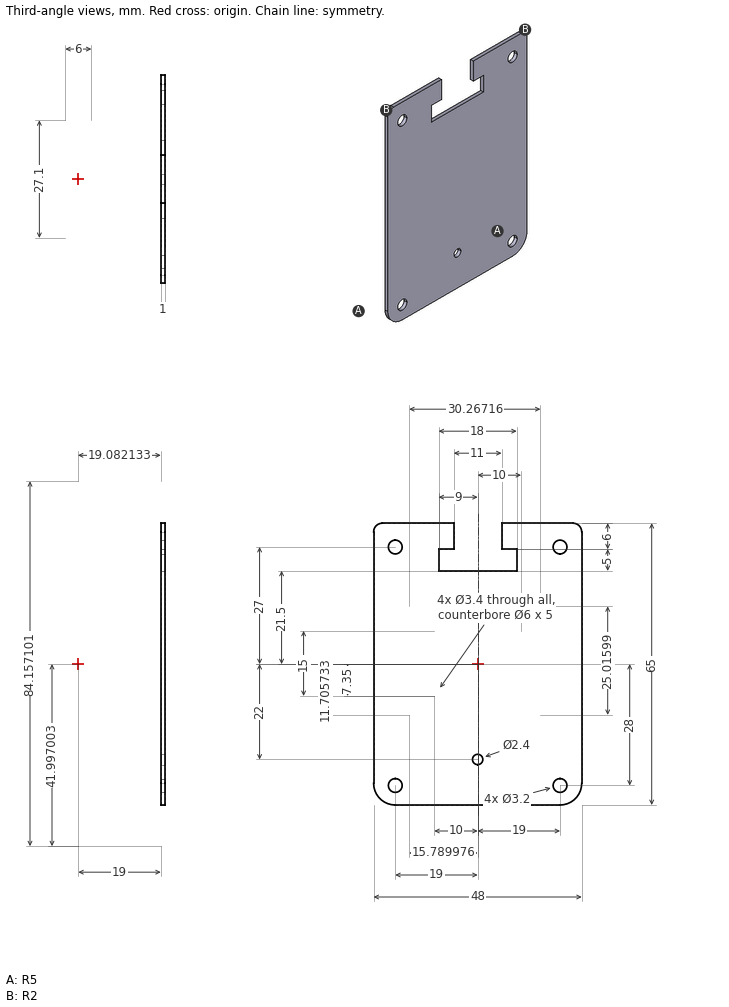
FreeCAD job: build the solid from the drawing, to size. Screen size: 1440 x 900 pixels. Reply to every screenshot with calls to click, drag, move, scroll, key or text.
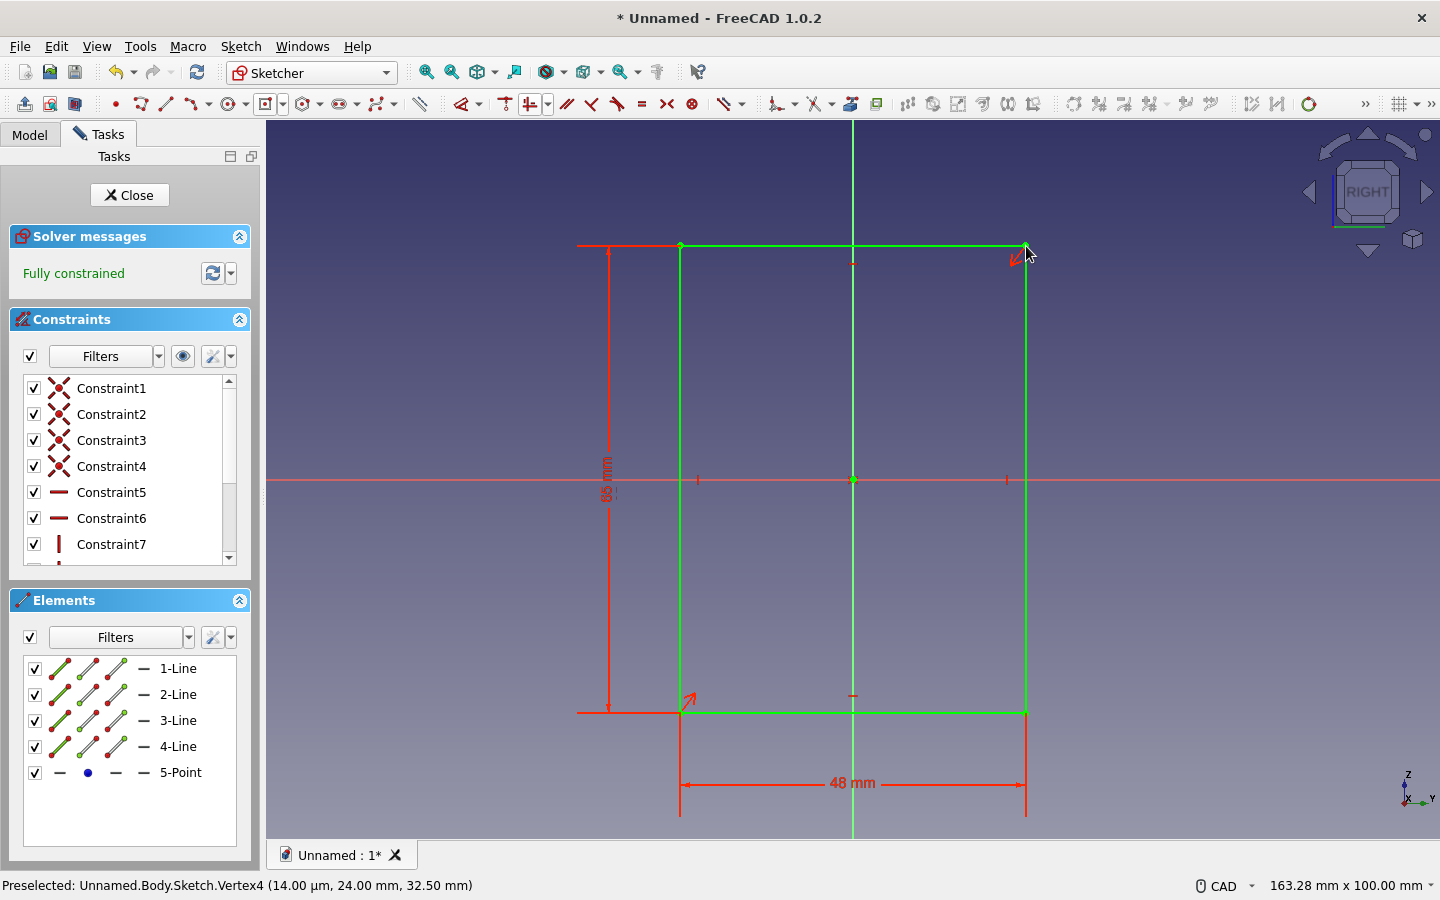
click(130, 195)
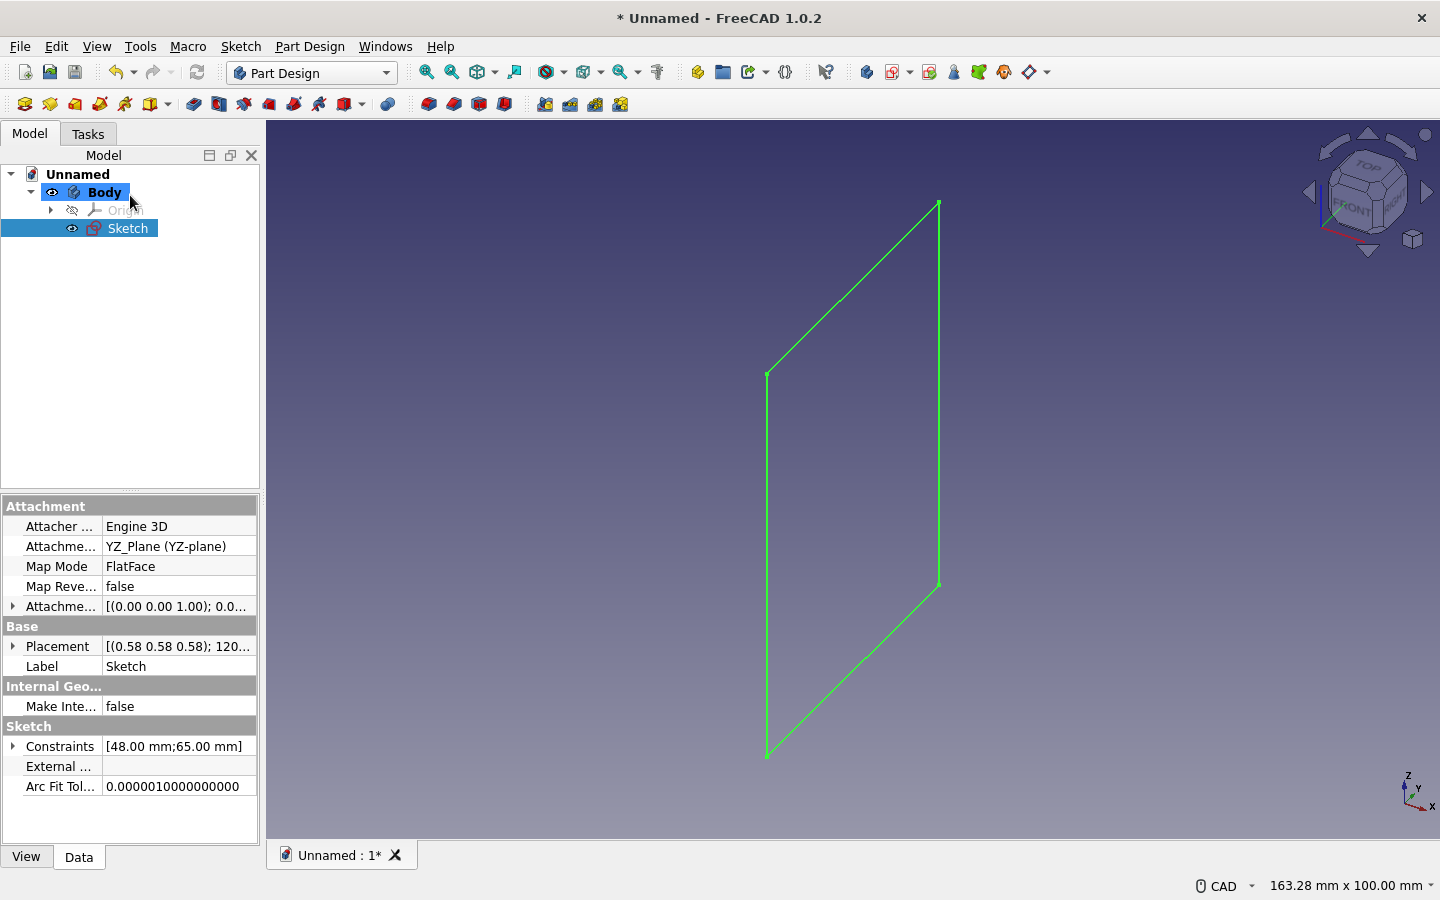
click(25, 104)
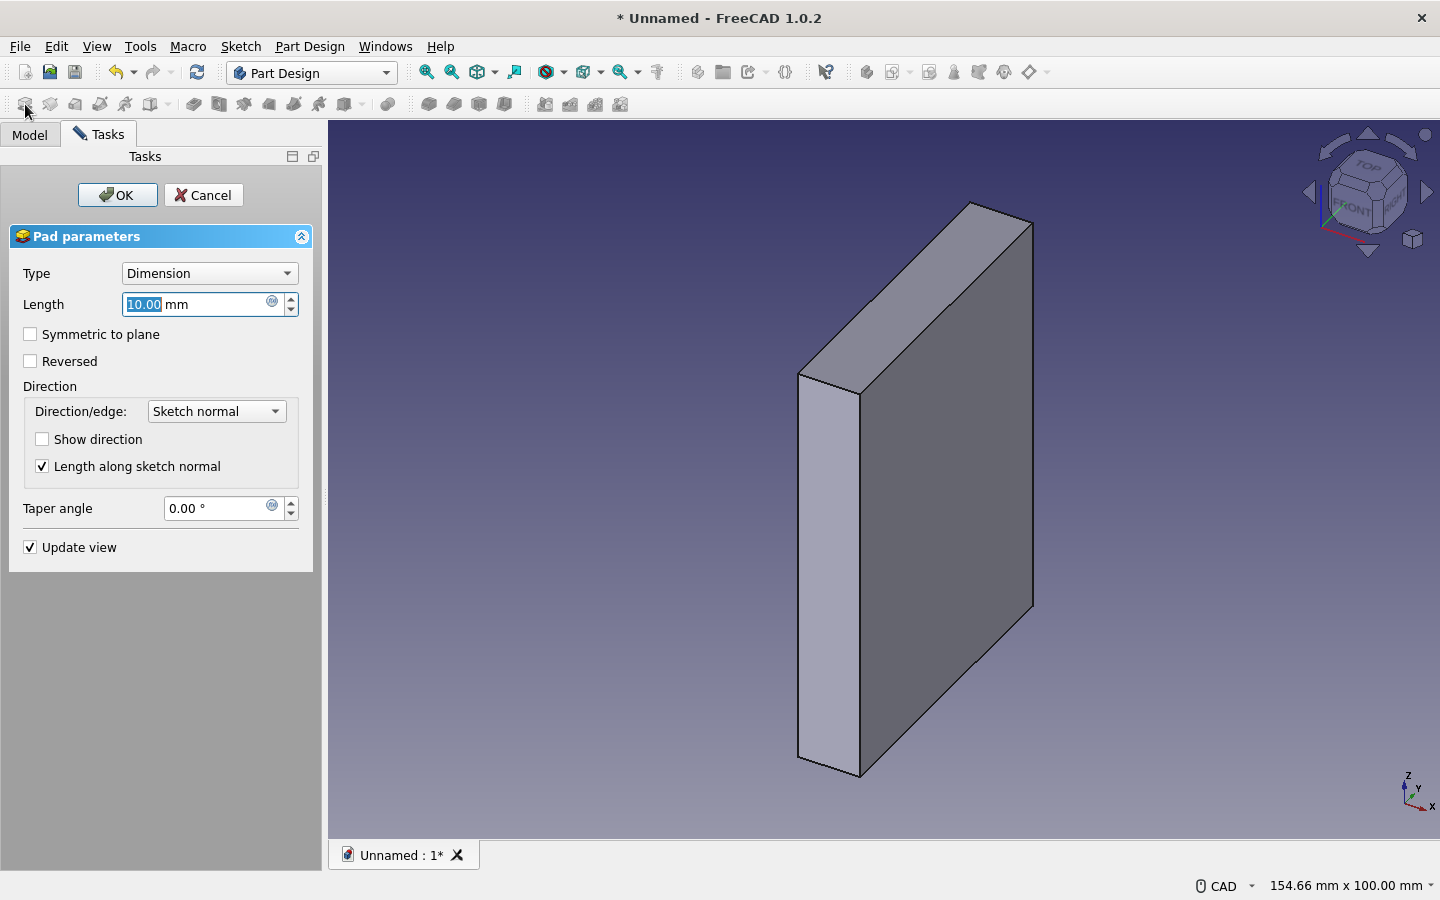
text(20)
key(Tab)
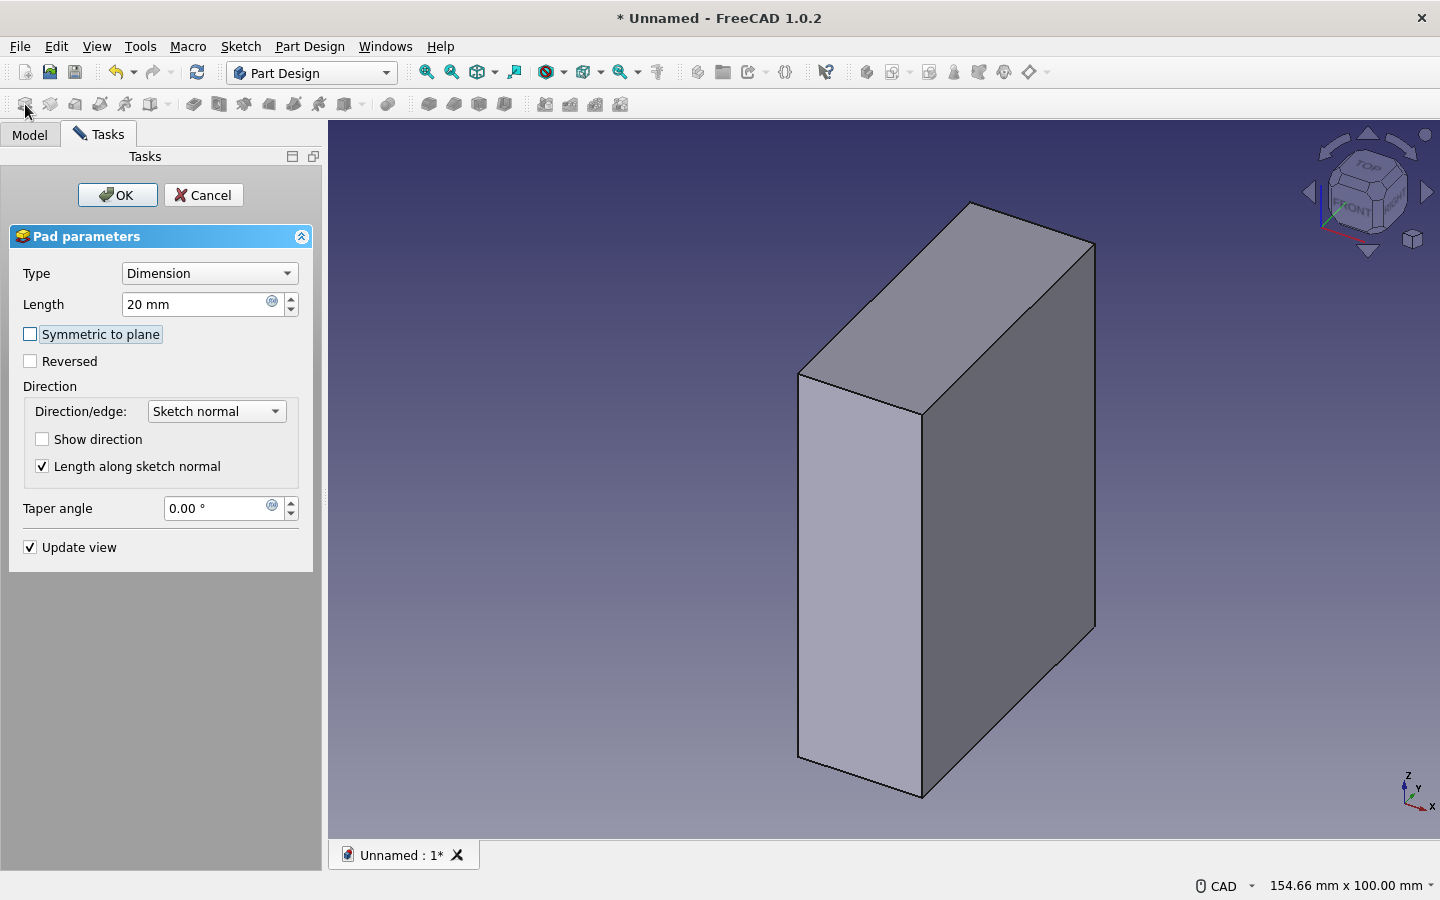
click(118, 195)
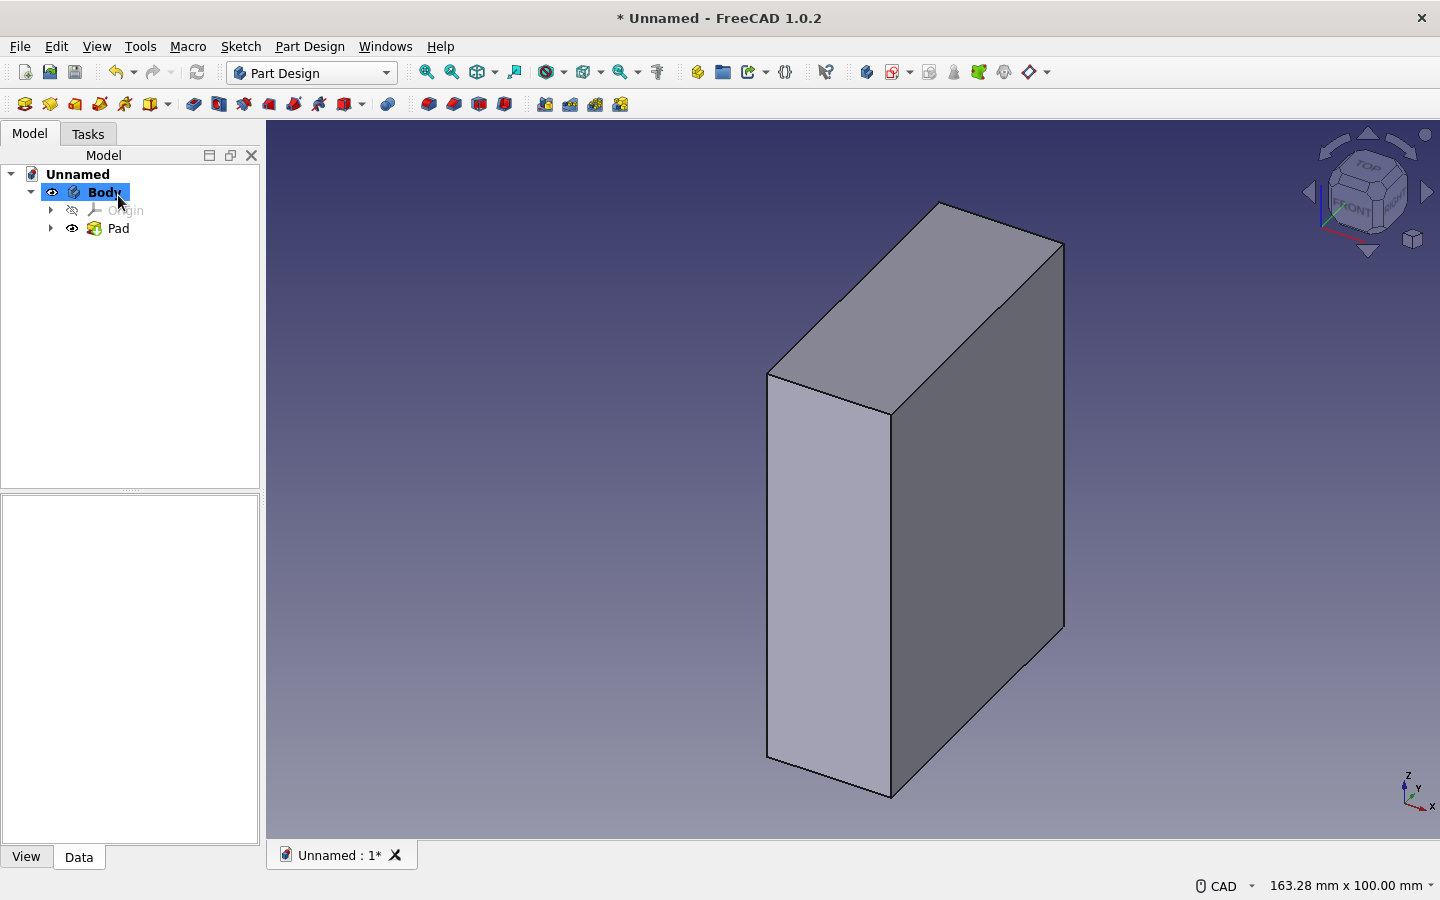
key(5)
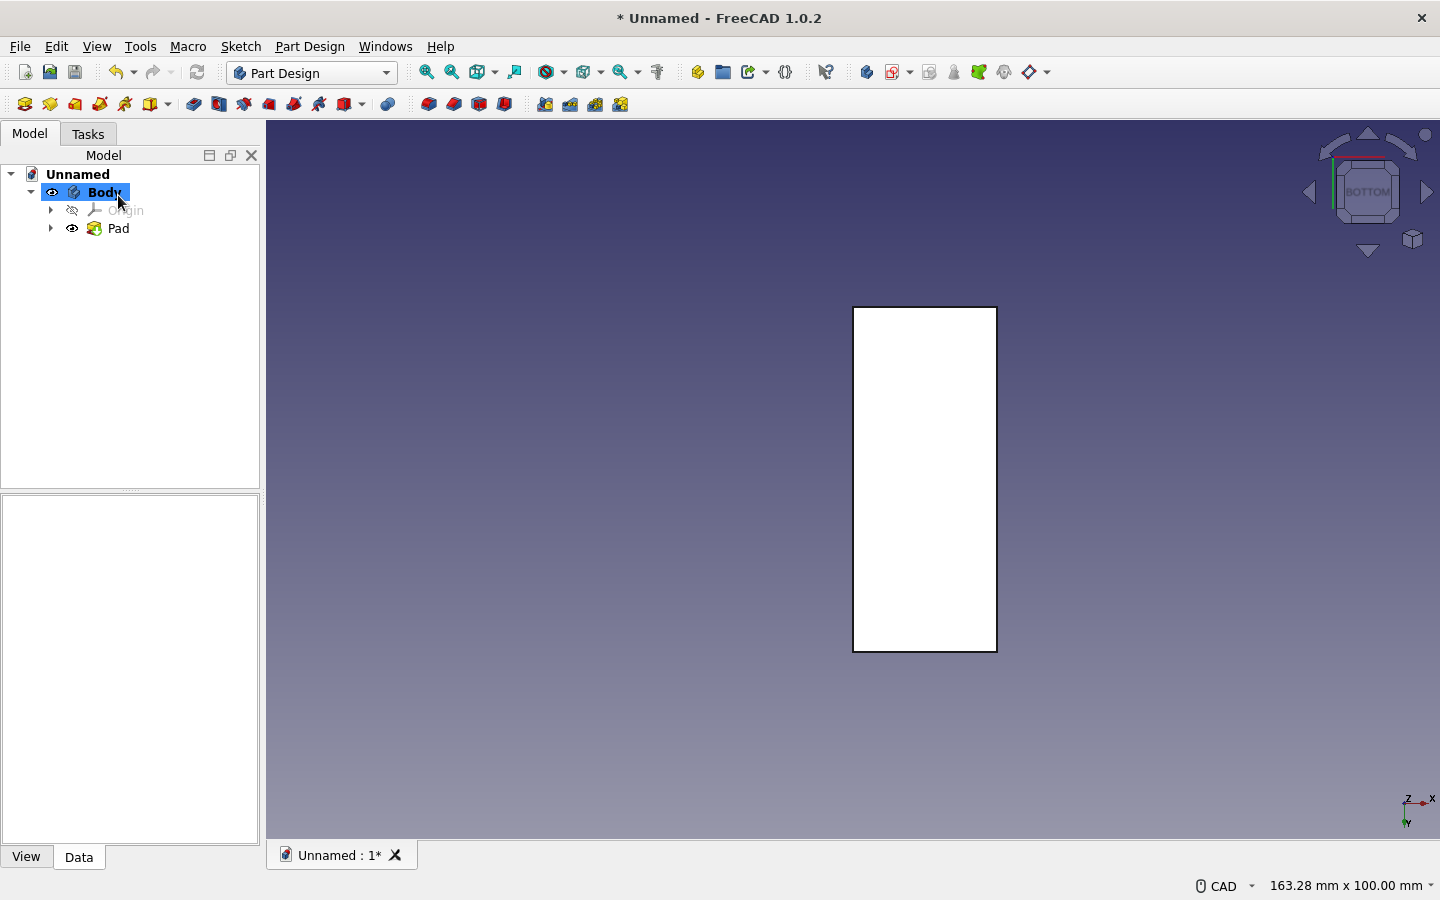
click(925, 577)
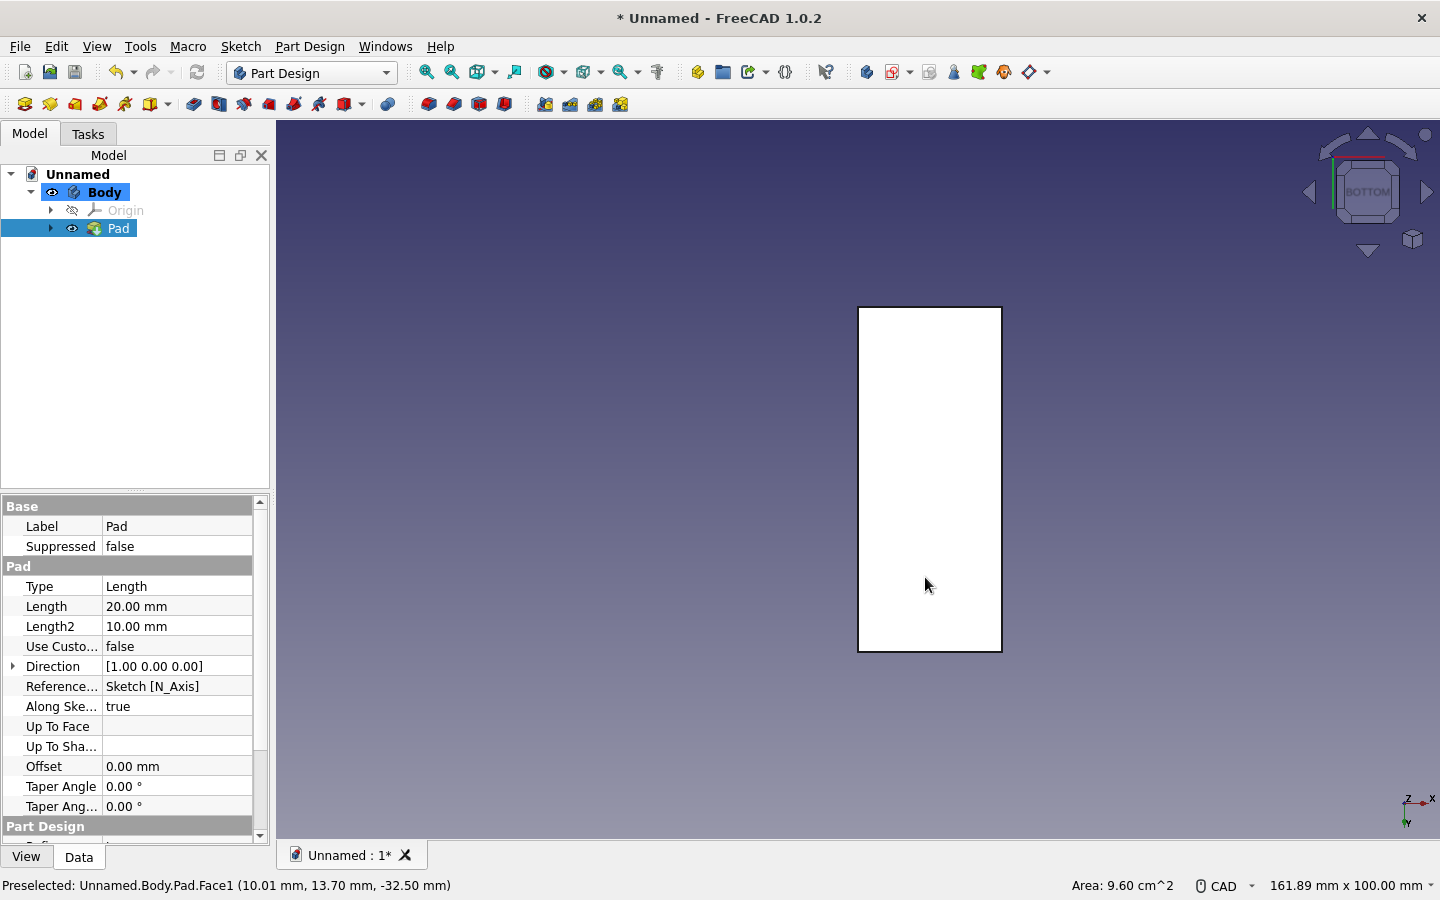
click(892, 72)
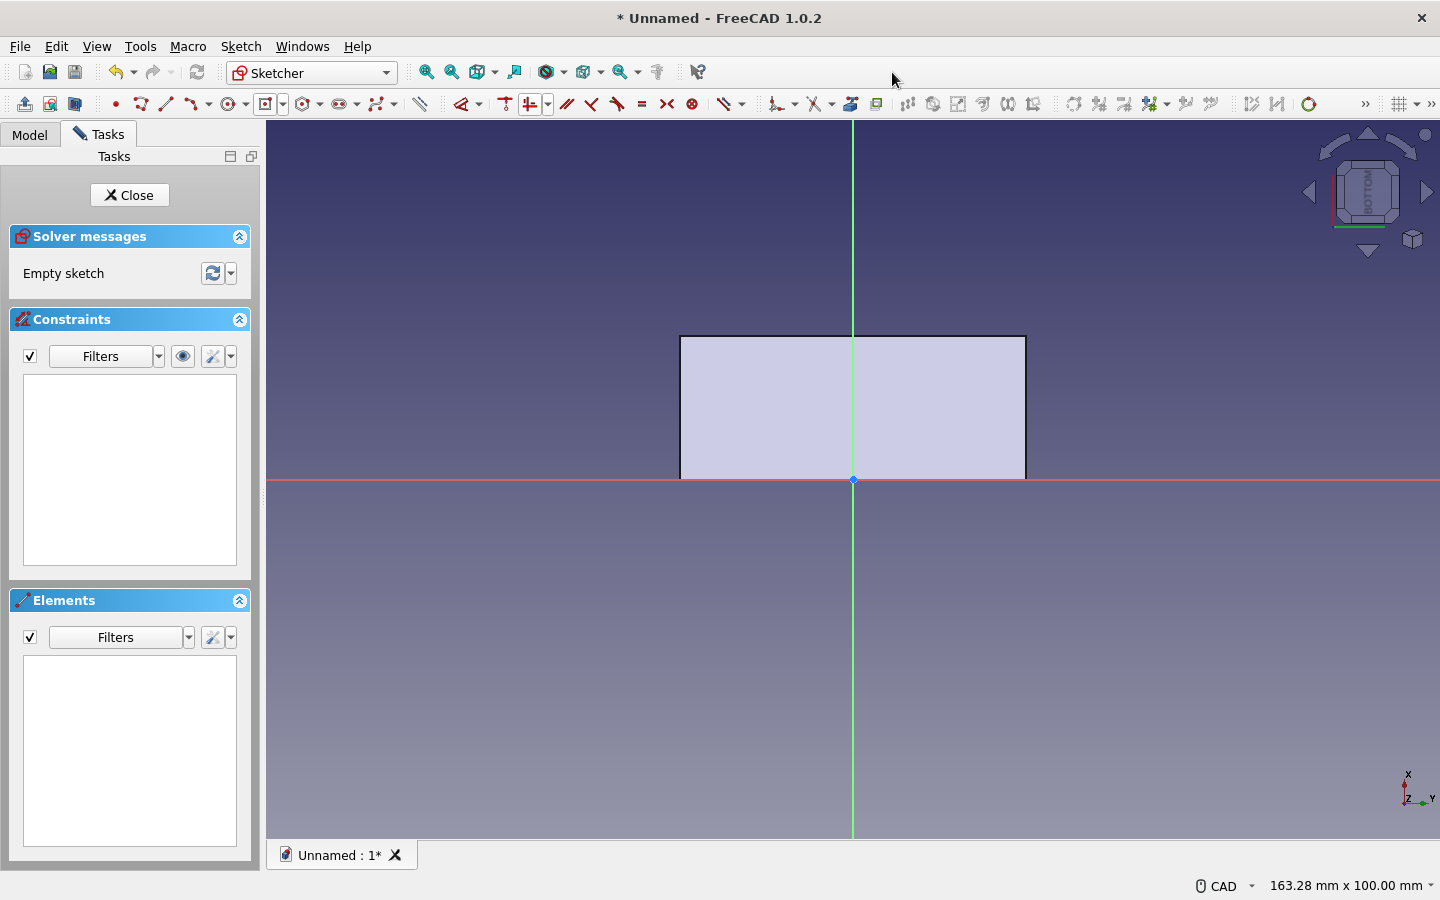
scroll(883, 480, up, 6)